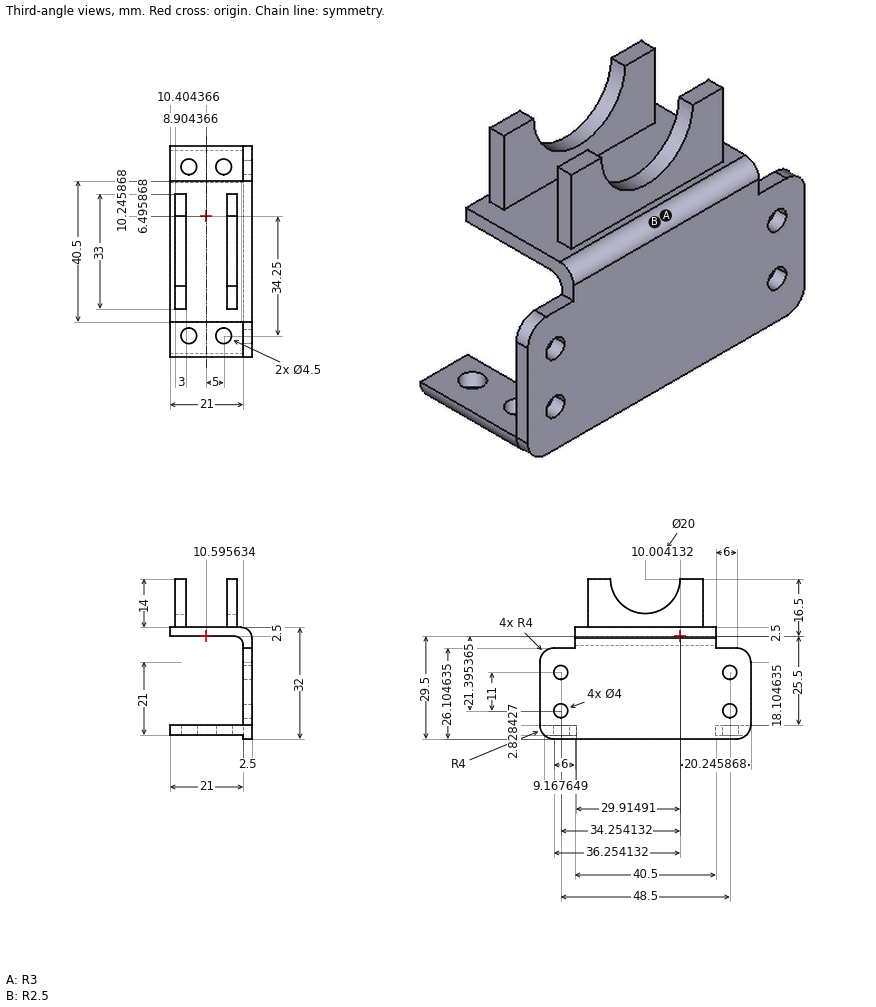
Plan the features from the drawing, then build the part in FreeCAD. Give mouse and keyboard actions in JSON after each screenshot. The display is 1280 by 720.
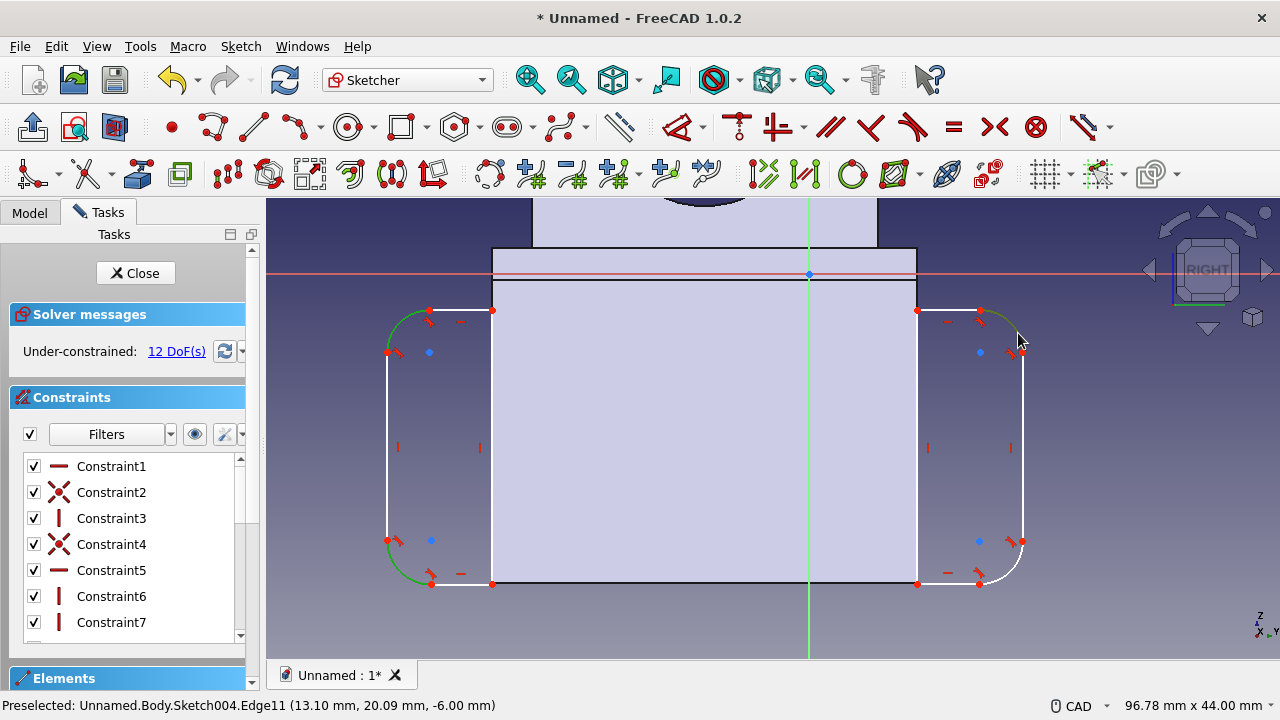
{"action": "left_click", "coordinate": [999, 579]}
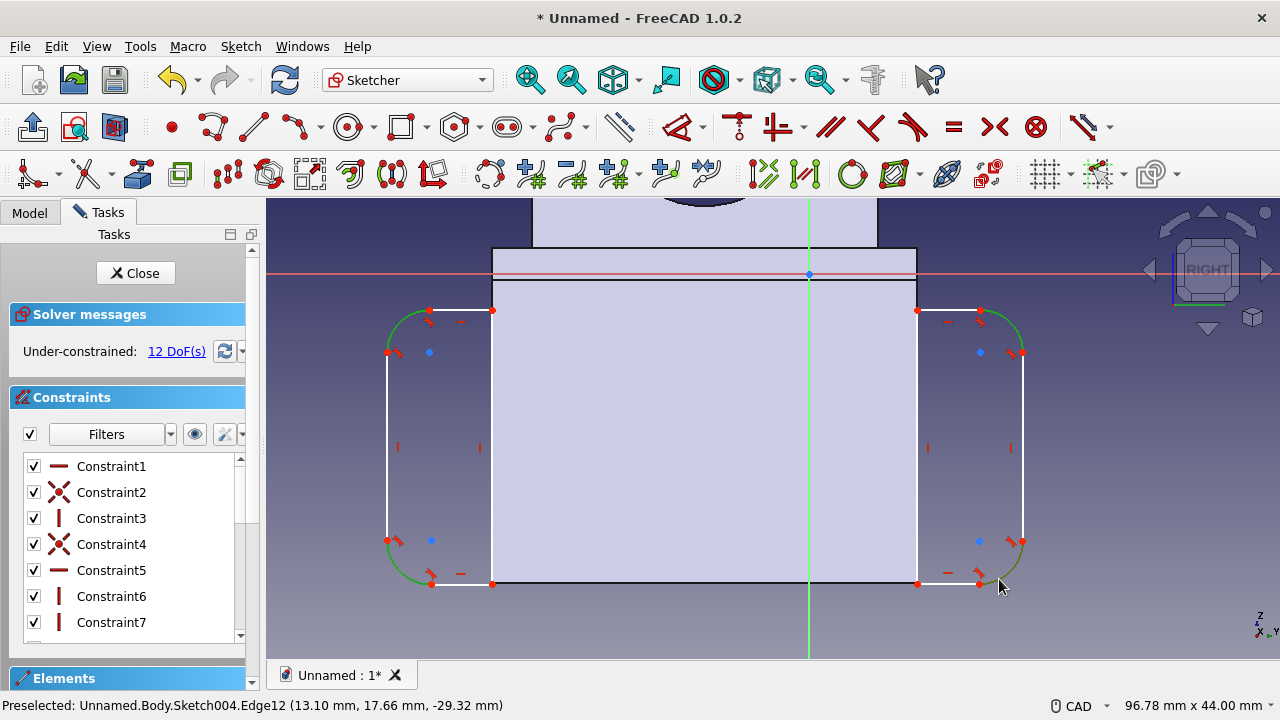
{"action": "left_click", "coordinate": [954, 128]}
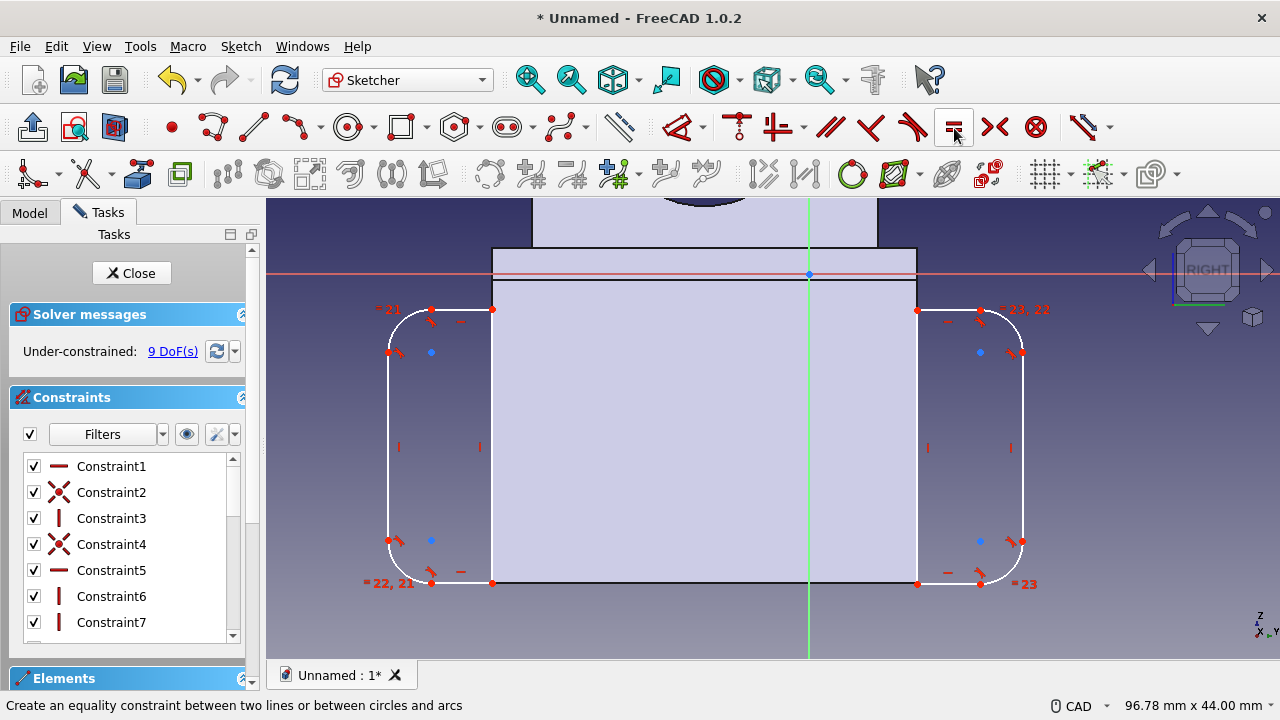
{"action": "left_click", "coordinate": [676, 128]}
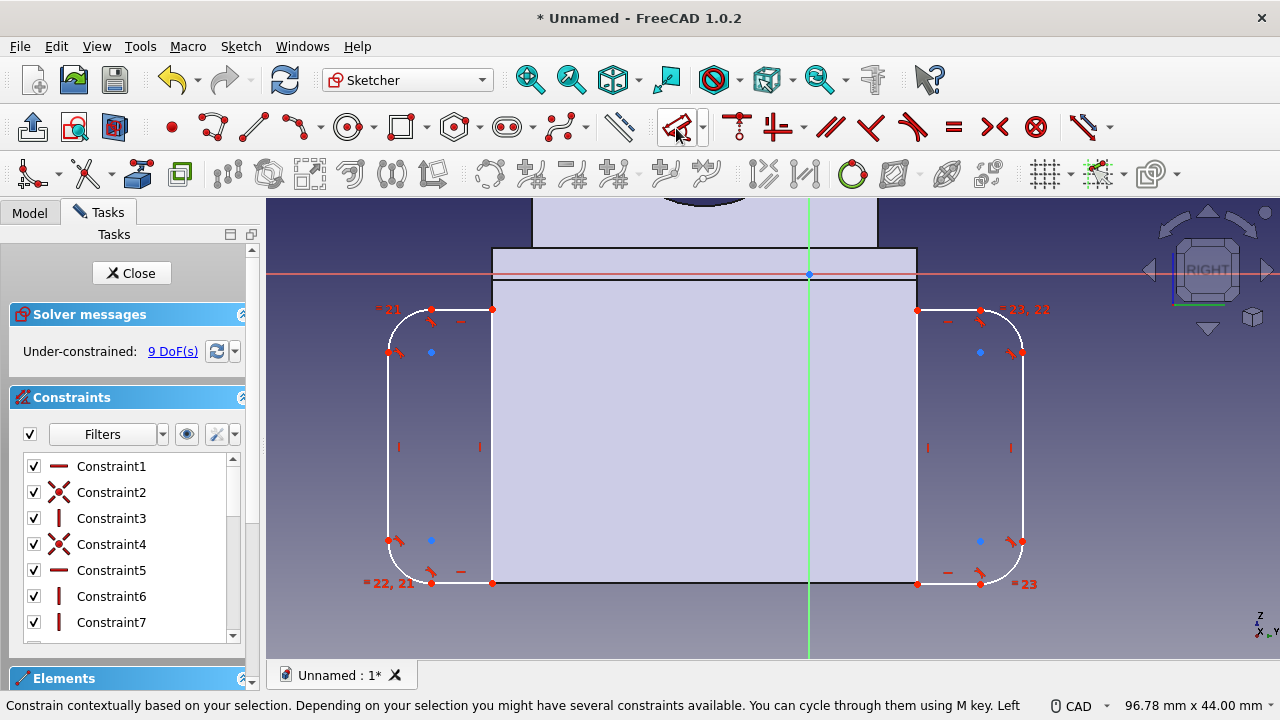
{"action": "left_click", "coordinate": [412, 315]}
{"action": "left_click", "coordinate": [370, 311]}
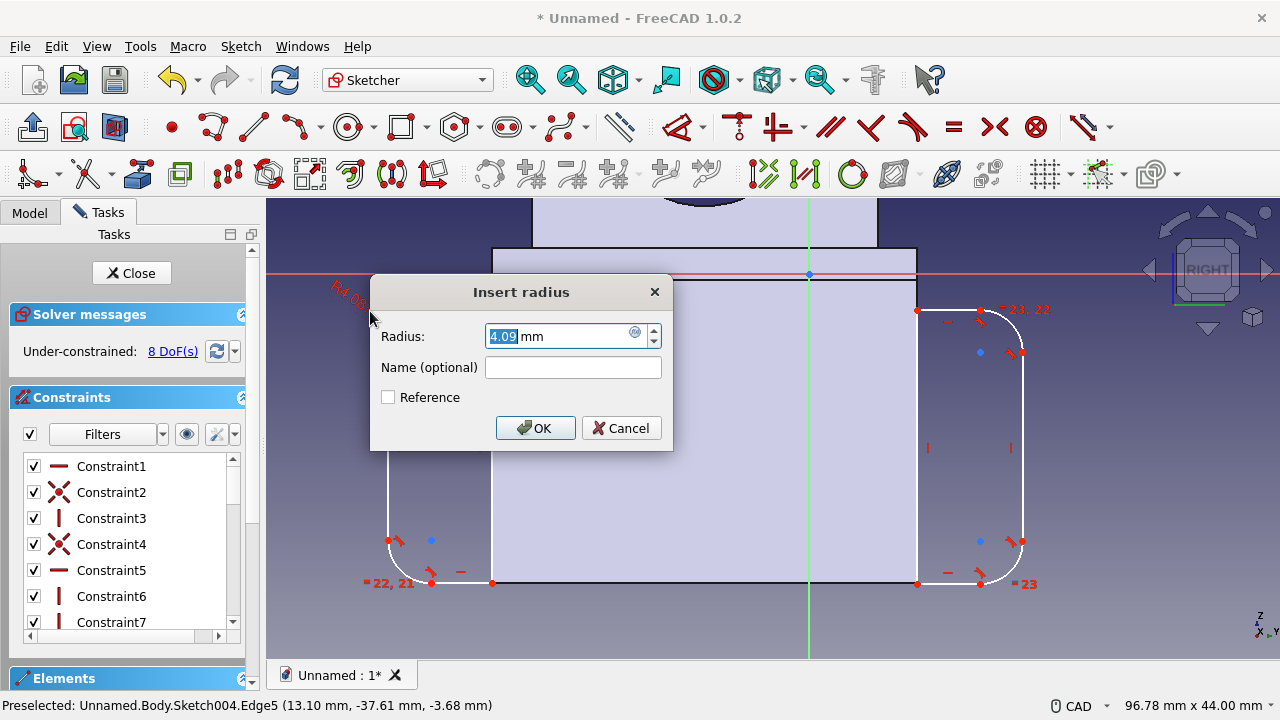
{"action": "type", "text": "4"}
{"action": "key", "text": "Return"}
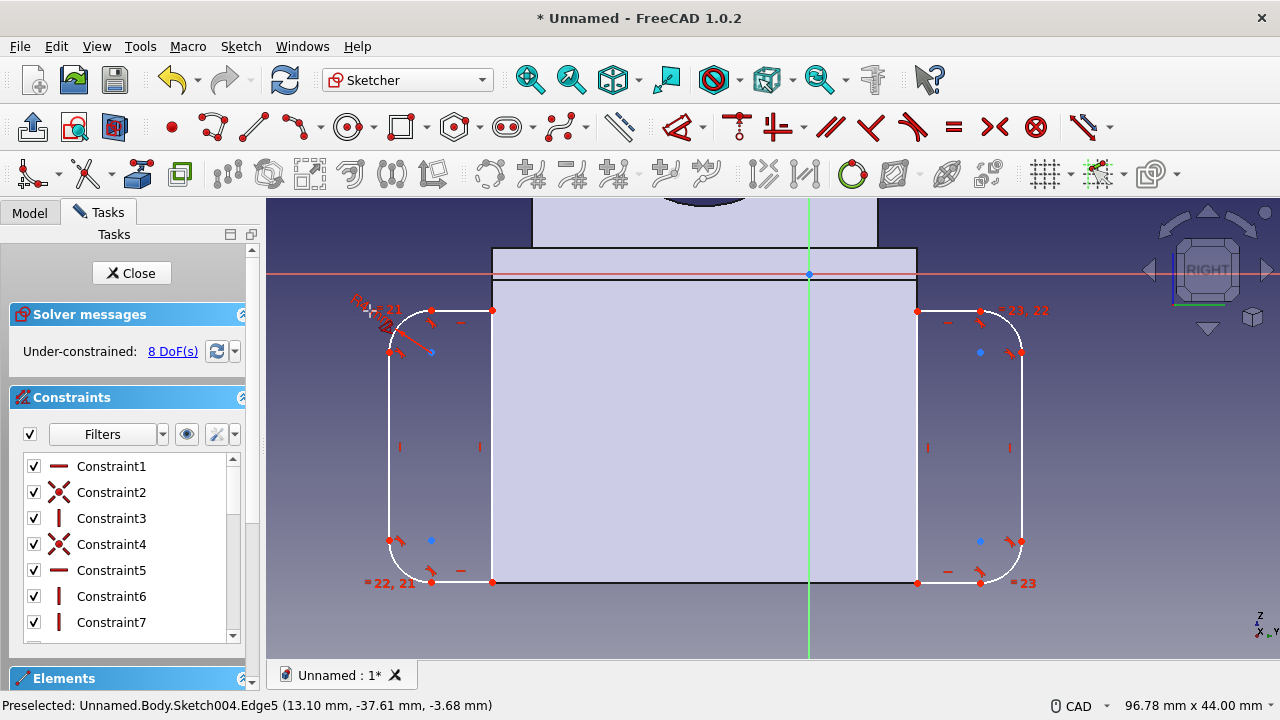
{"action": "left_click", "coordinate": [450, 582]}
{"action": "left_click", "coordinate": [462, 616]}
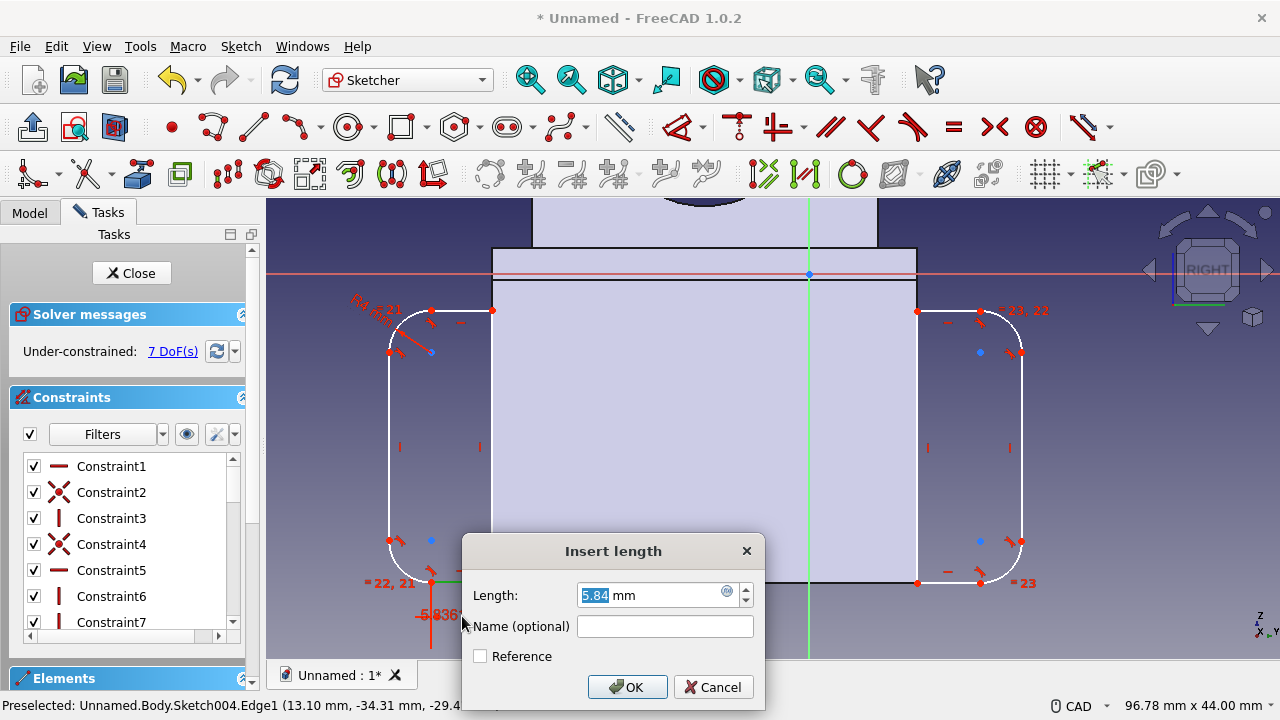
{"action": "type", "text": "6"}
{"action": "key", "text": "Return"}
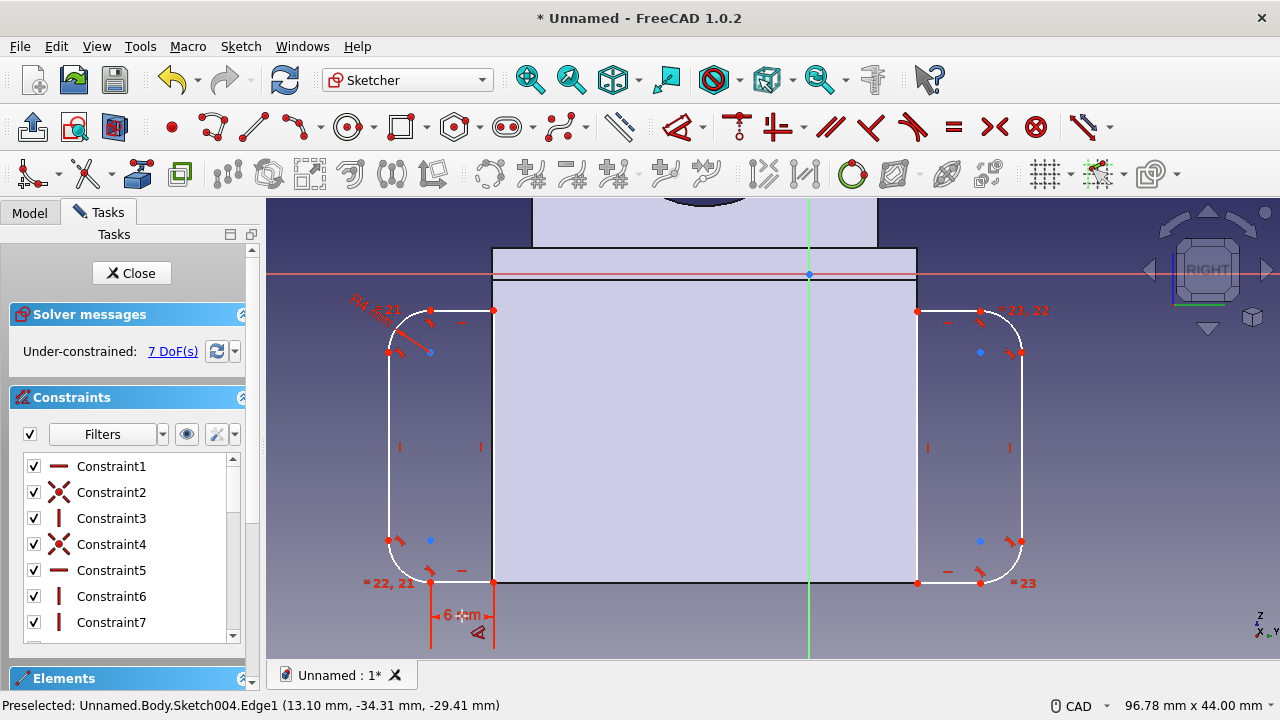
{"action": "left_click", "coordinate": [961, 311]}
{"action": "left_click", "coordinate": [948, 345]}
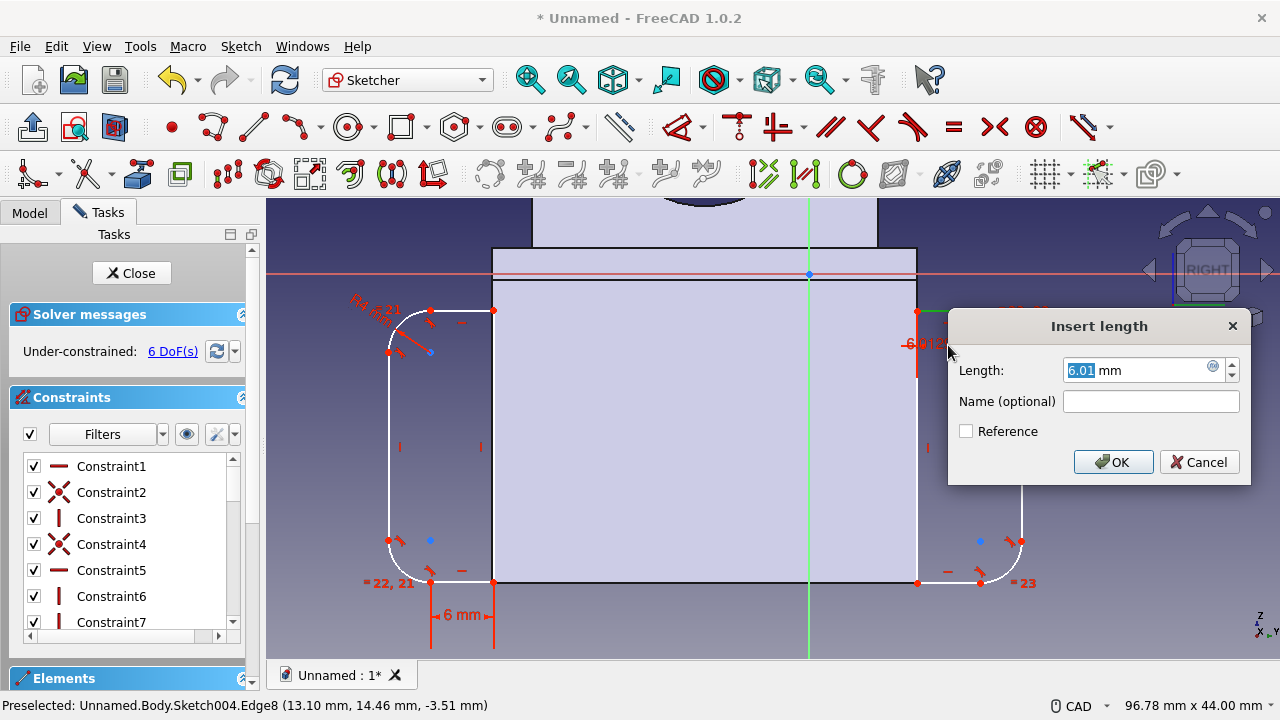
{"action": "type", "text": "6"}
{"action": "key", "text": "Return"}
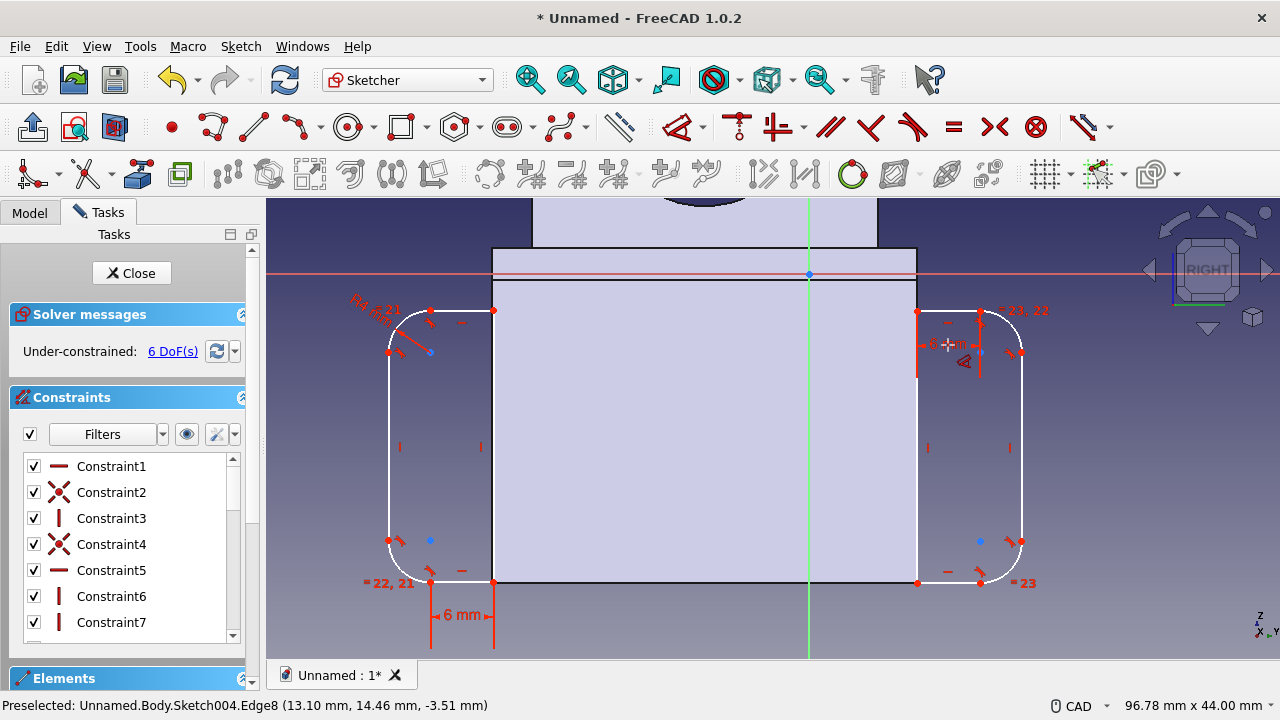
{"action": "left_click", "coordinate": [431, 582]}
{"action": "left_click", "coordinate": [843, 428]}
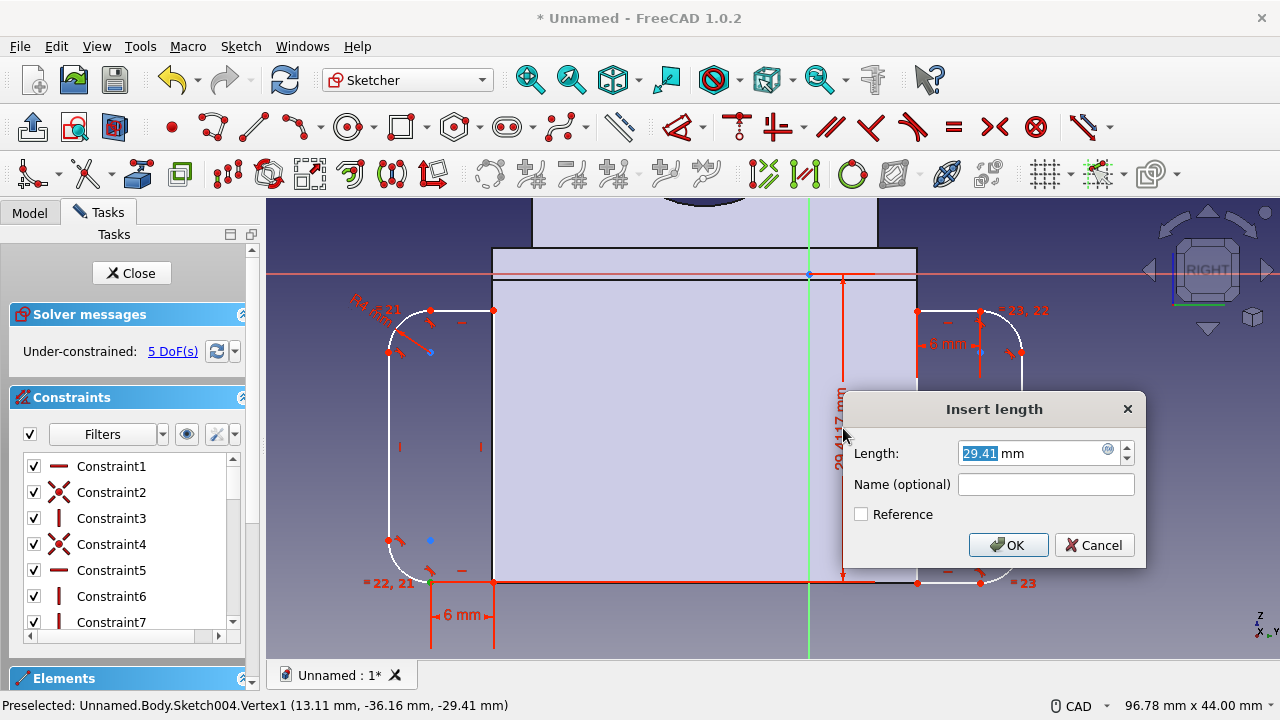
{"action": "type", "text": "29.5"}
{"action": "key", "text": "Return"}